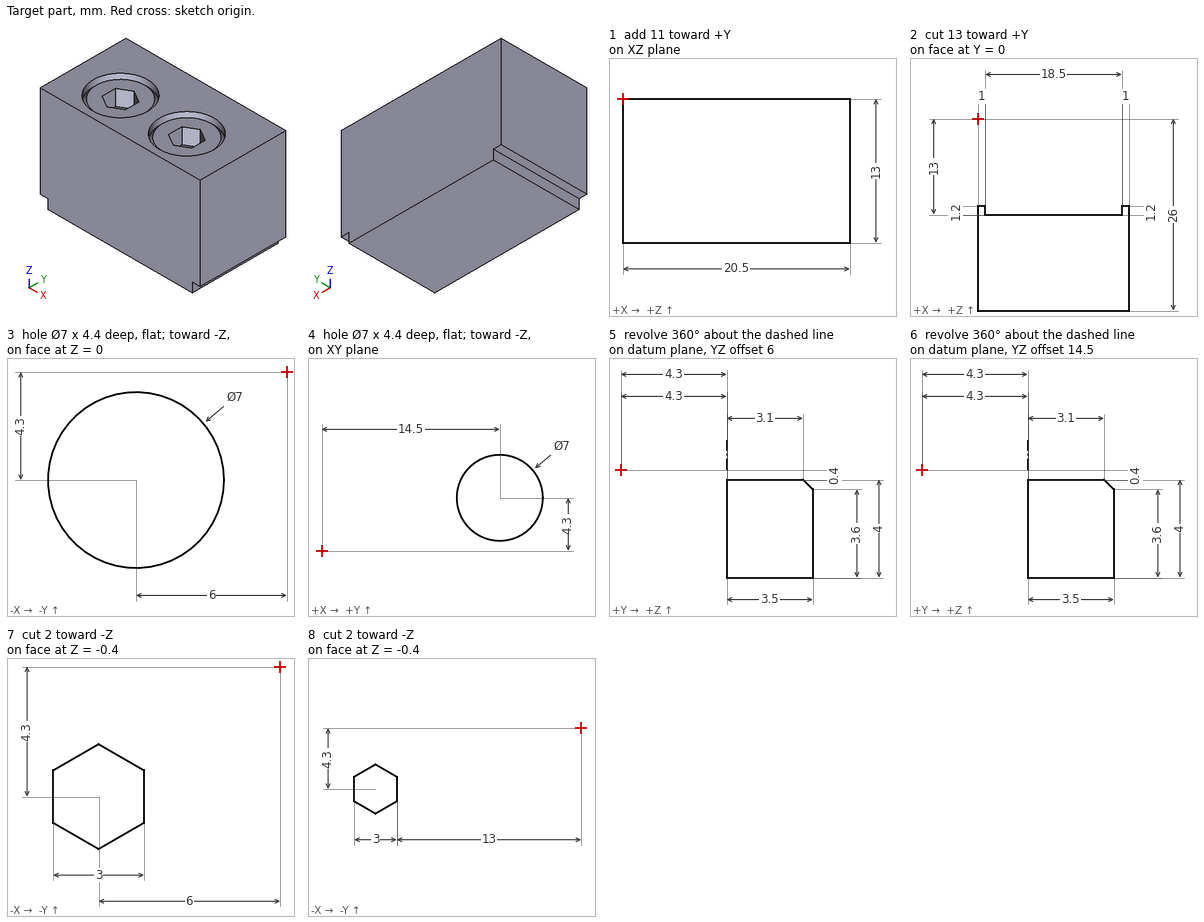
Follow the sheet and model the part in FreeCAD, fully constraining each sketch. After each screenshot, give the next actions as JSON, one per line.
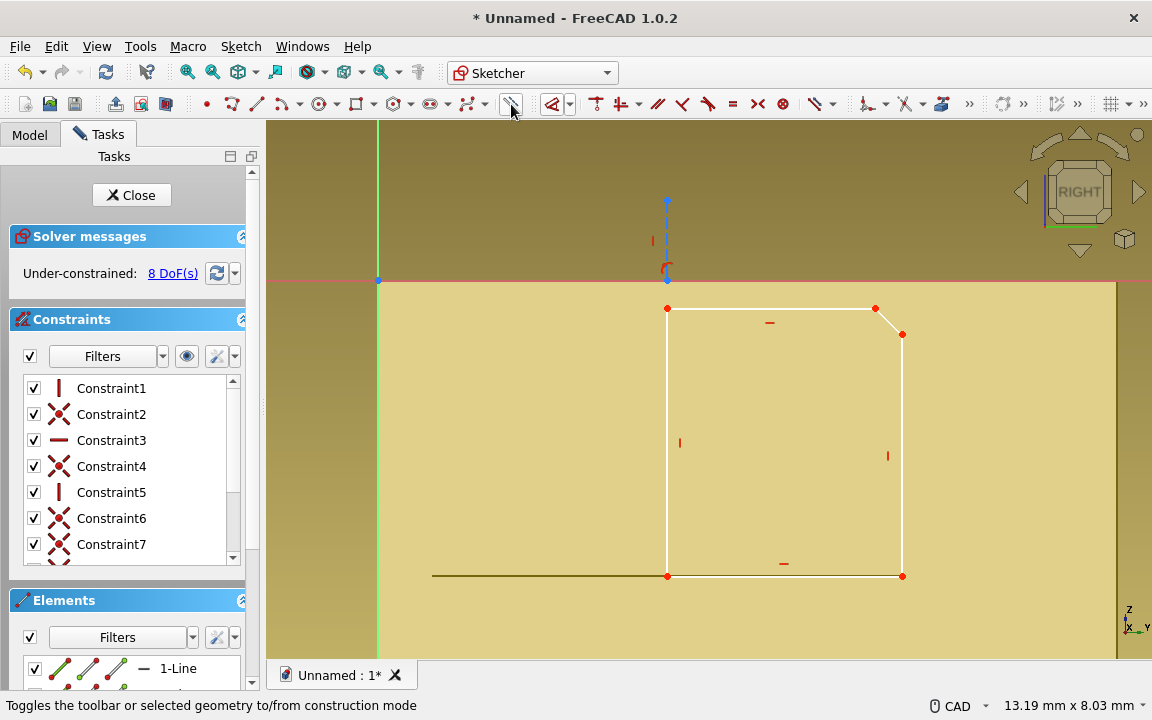
{"action": "left_click", "coordinate": [667, 389]}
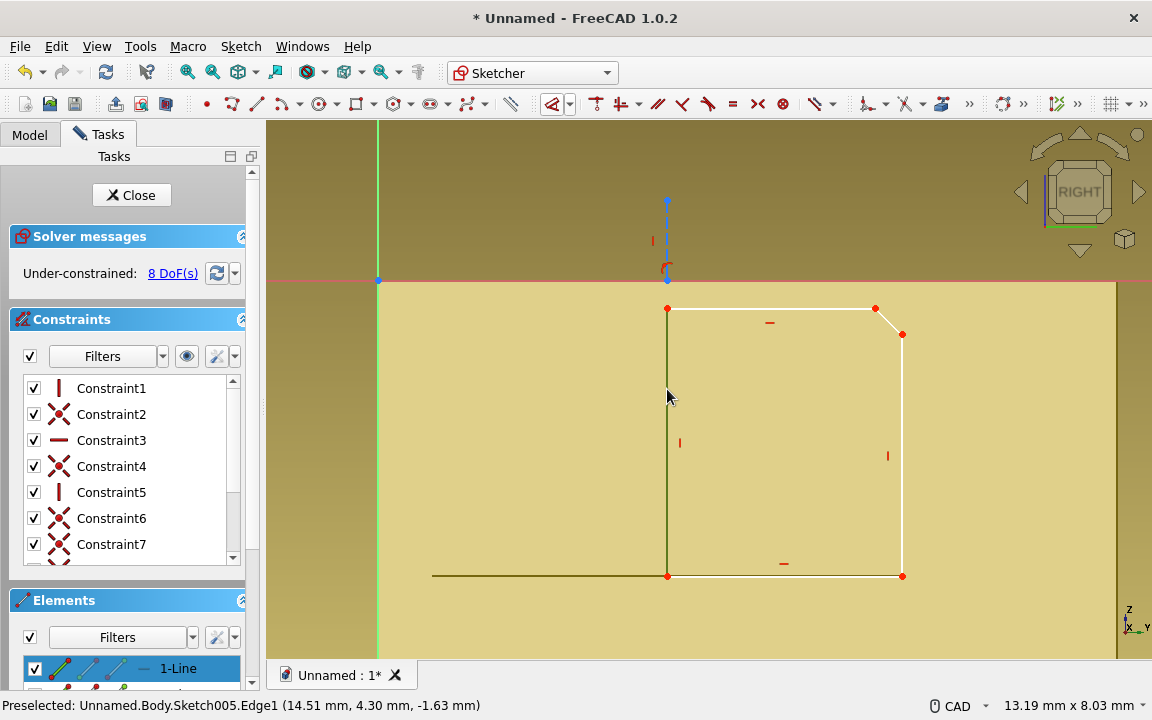
{"action": "key", "text": "i"}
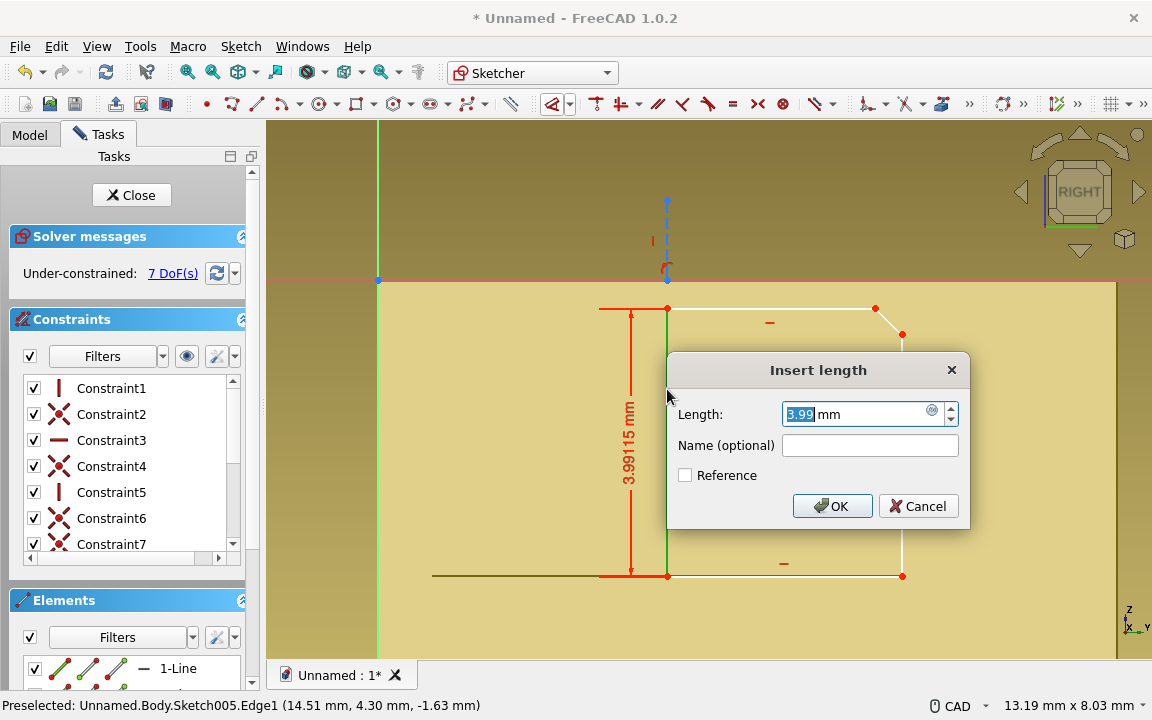
{"action": "type", "text": "4"}
{"action": "key", "text": "Return"}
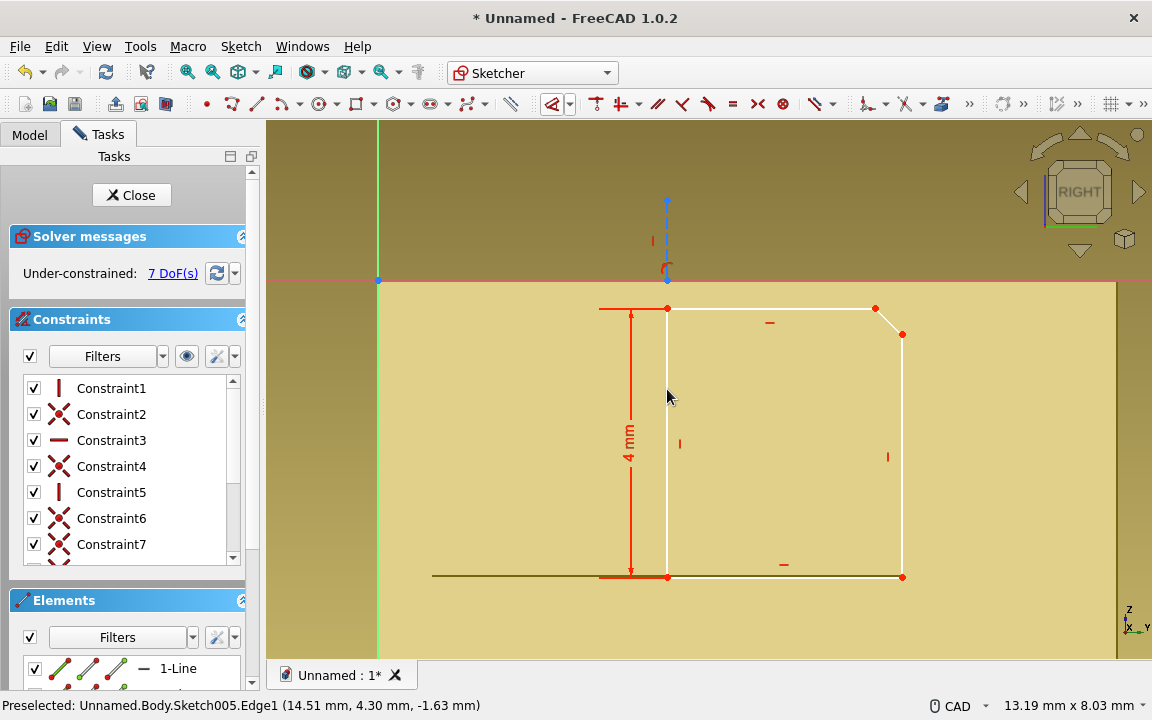
{"action": "left_click", "coordinate": [738, 578]}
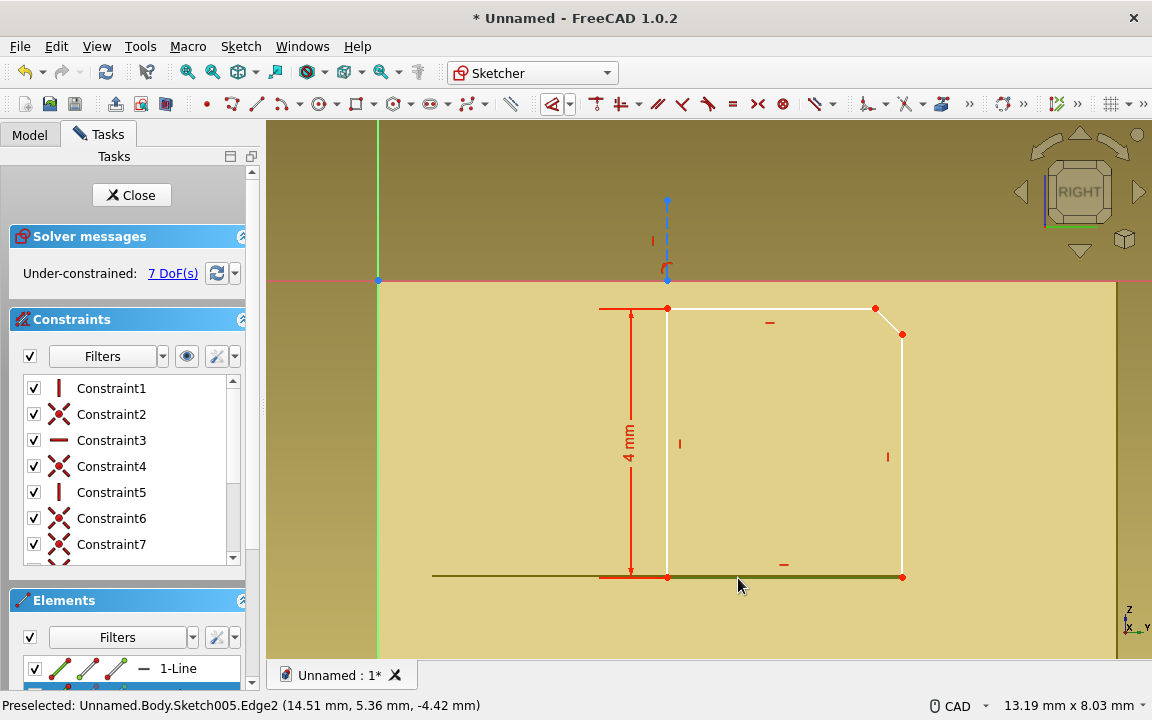
{"action": "key", "text": "l"}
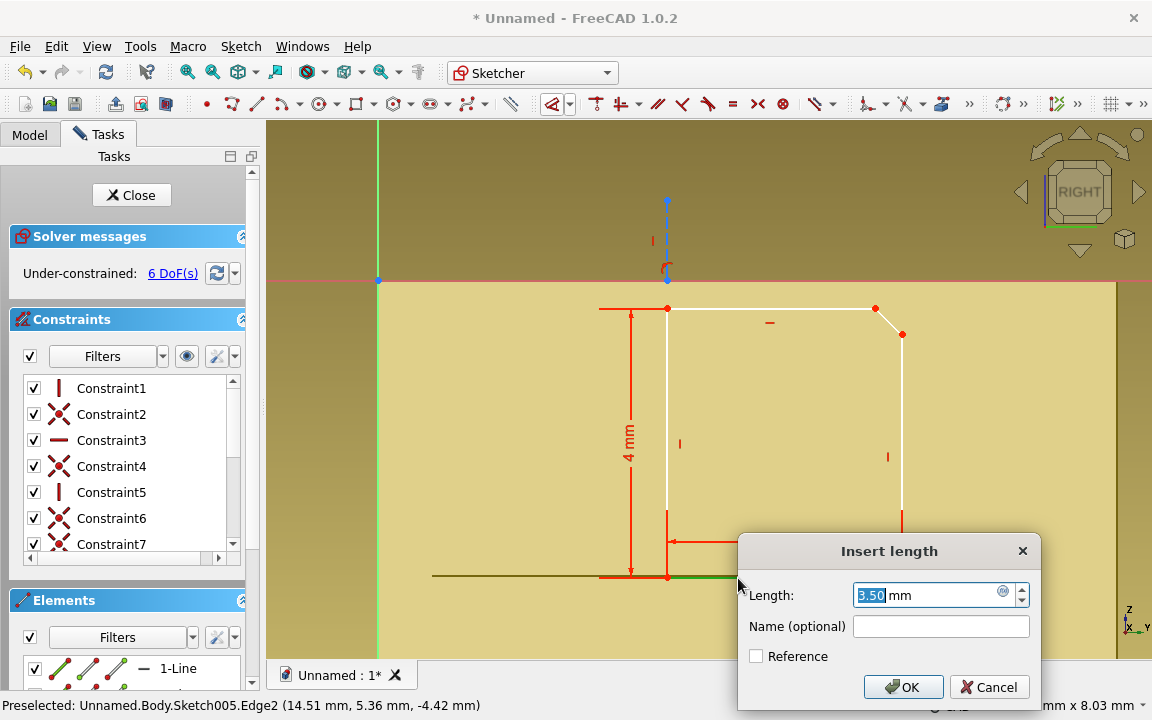
{"action": "type", "text": "3.5"}
{"action": "key", "text": "Return"}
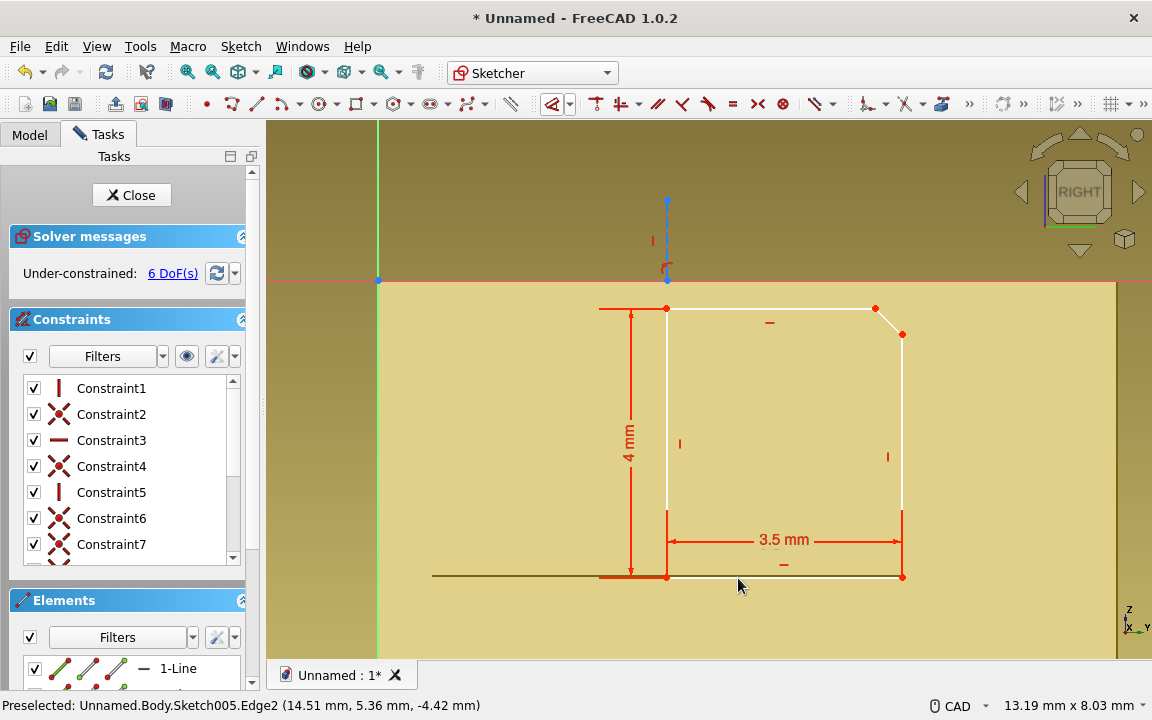
{"action": "left_click", "coordinate": [902, 505]}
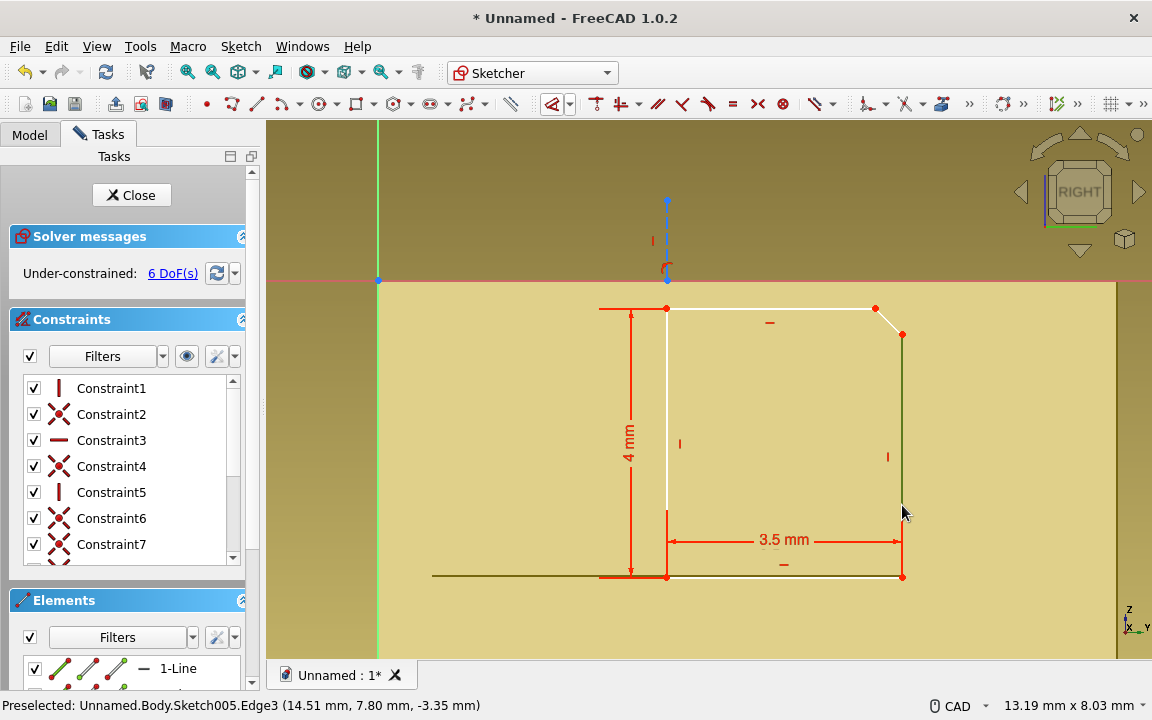
{"action": "left_click", "coordinate": [570, 104]}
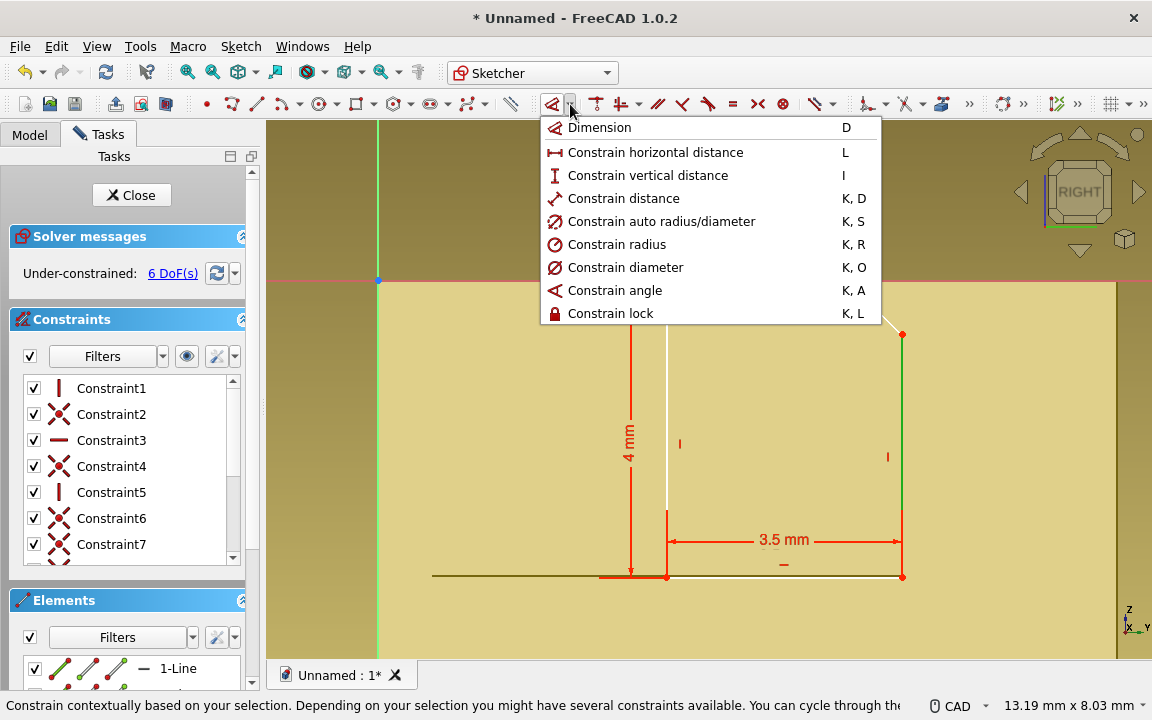
{"action": "left_click", "coordinate": [711, 176]}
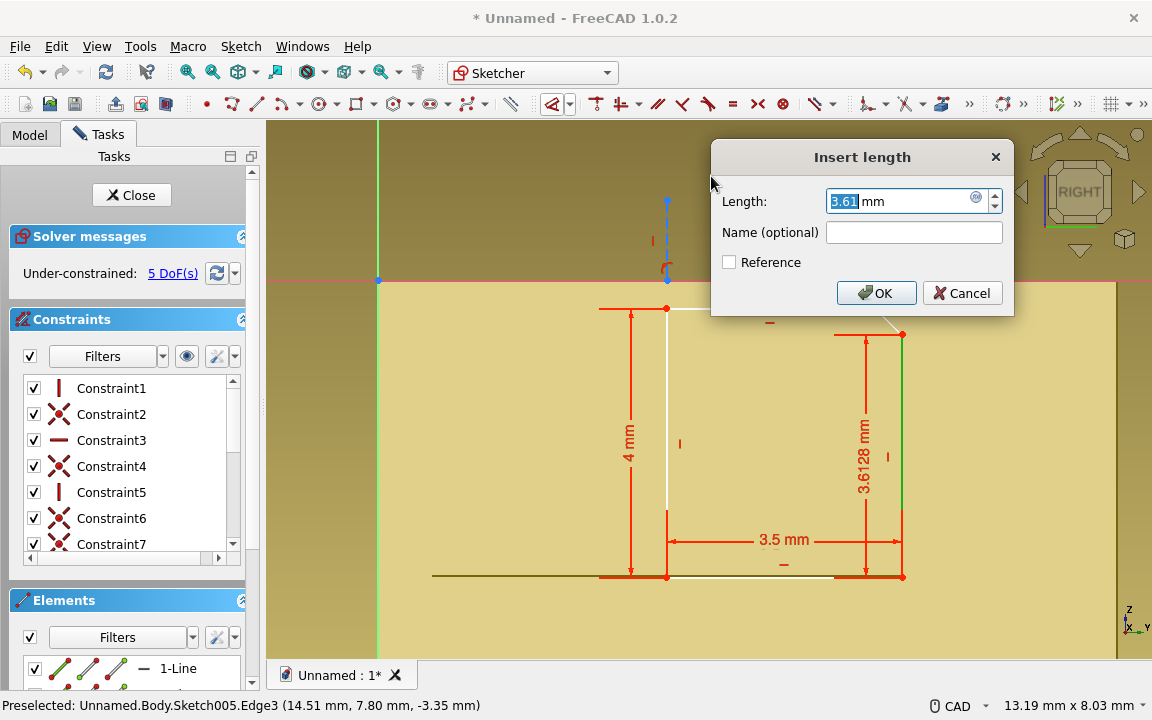
{"action": "type", "text": "3.6"}
{"action": "key", "text": "Return"}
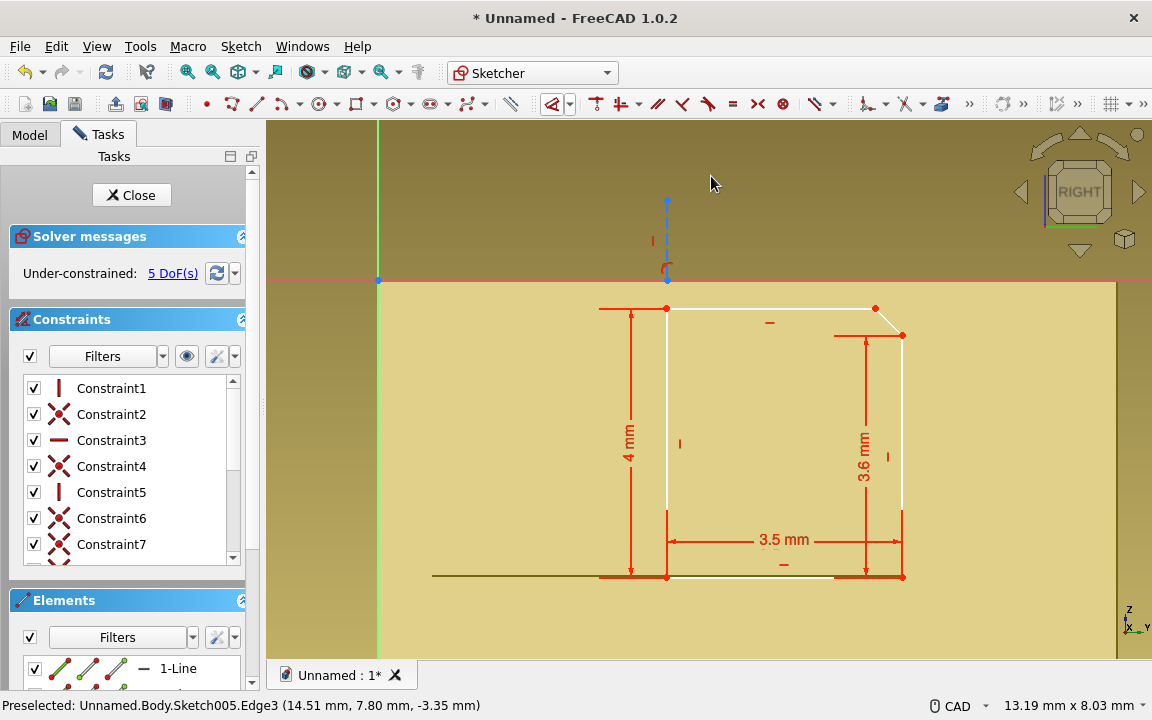
{"action": "left_click", "coordinate": [813, 309]}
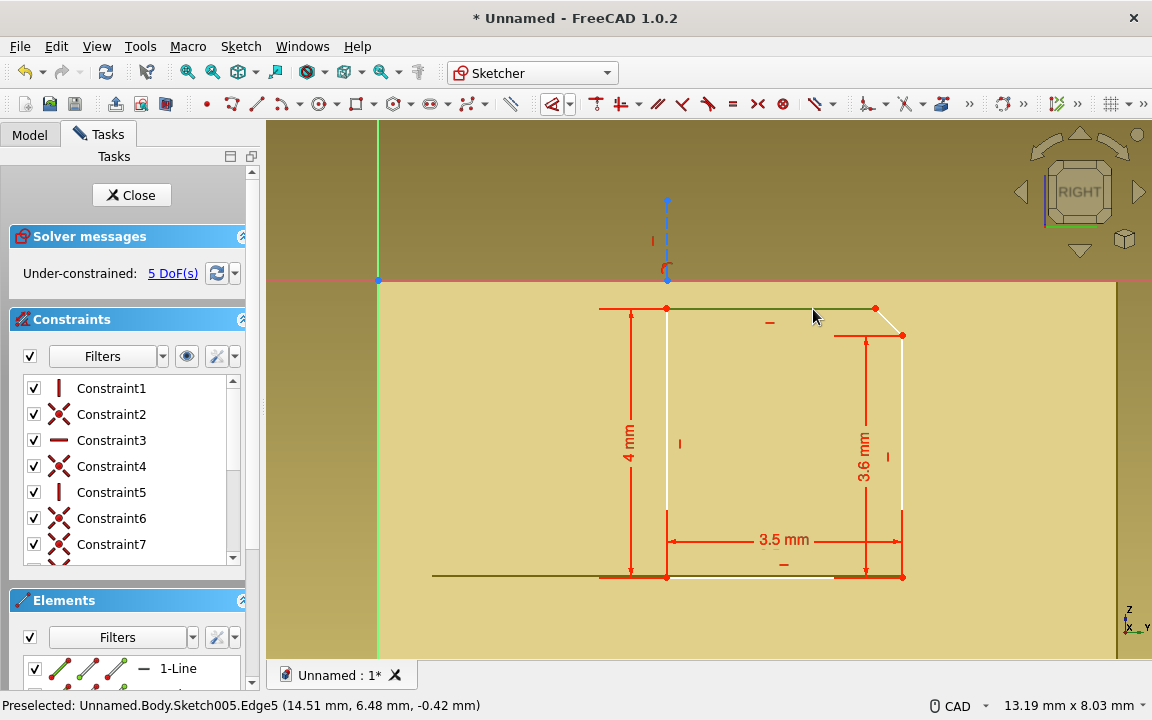
{"action": "left_click", "coordinate": [570, 104]}